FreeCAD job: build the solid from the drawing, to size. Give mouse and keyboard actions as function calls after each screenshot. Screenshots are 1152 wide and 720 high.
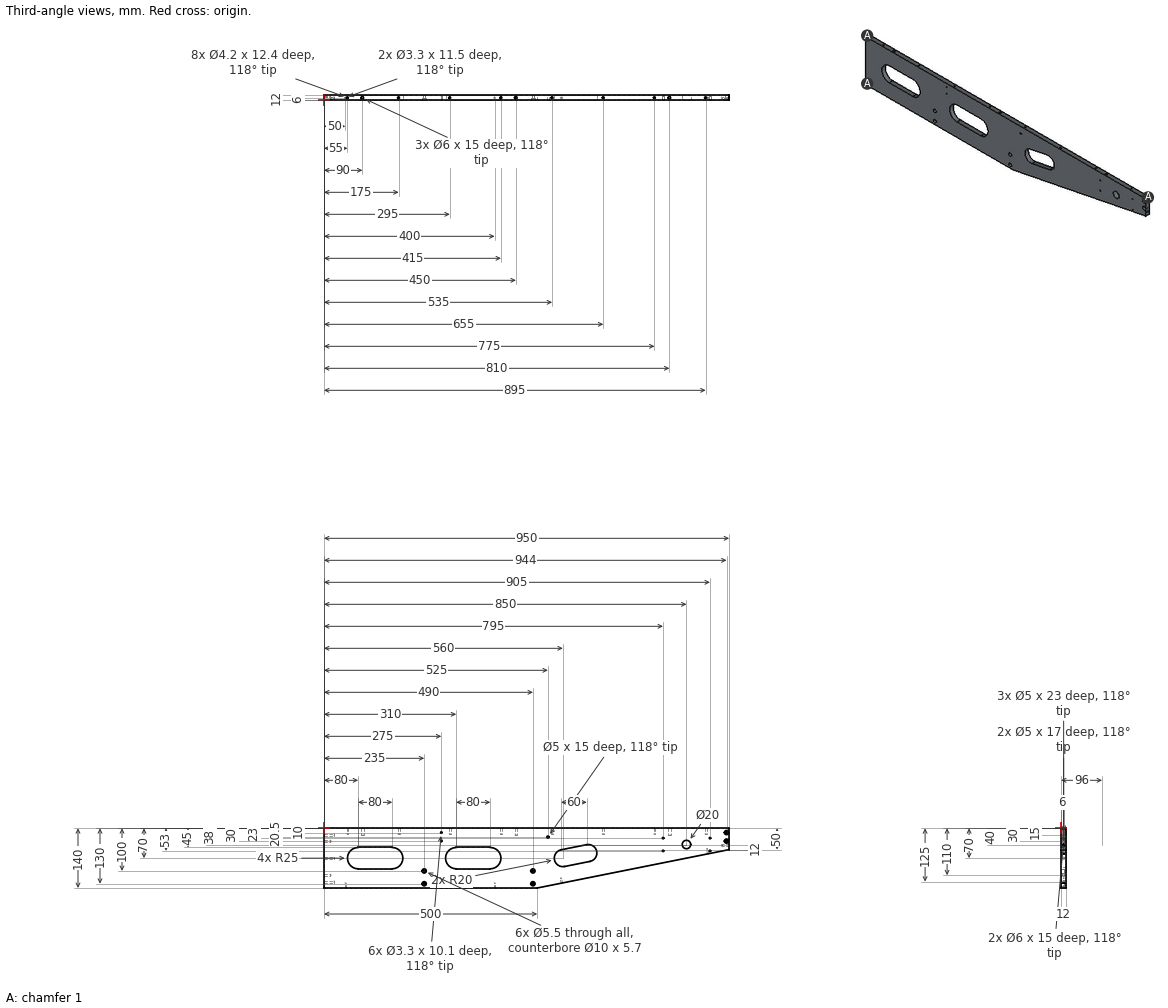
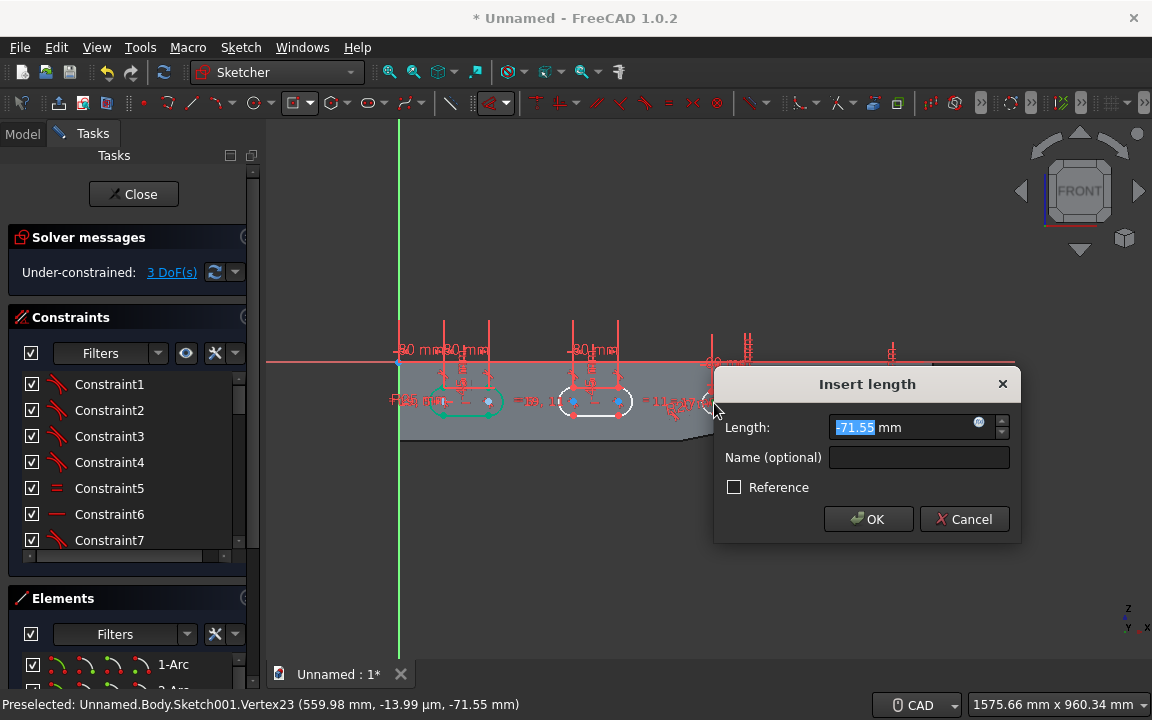
text(-70)
key(Return)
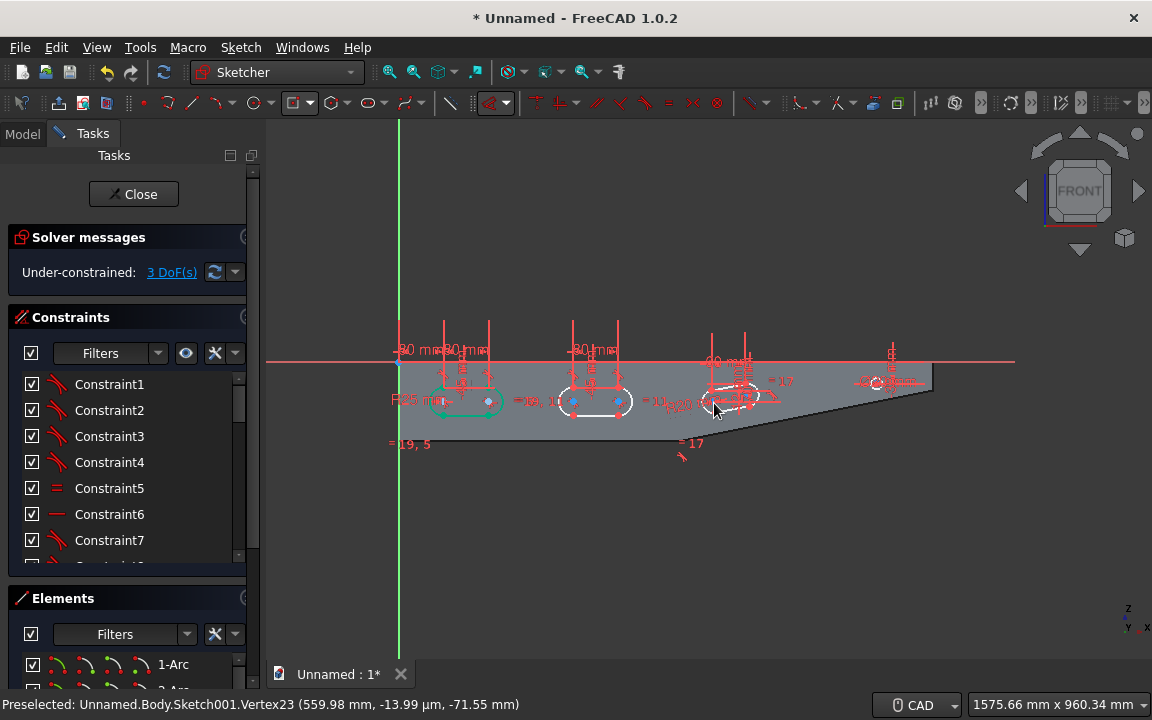
click(877, 384)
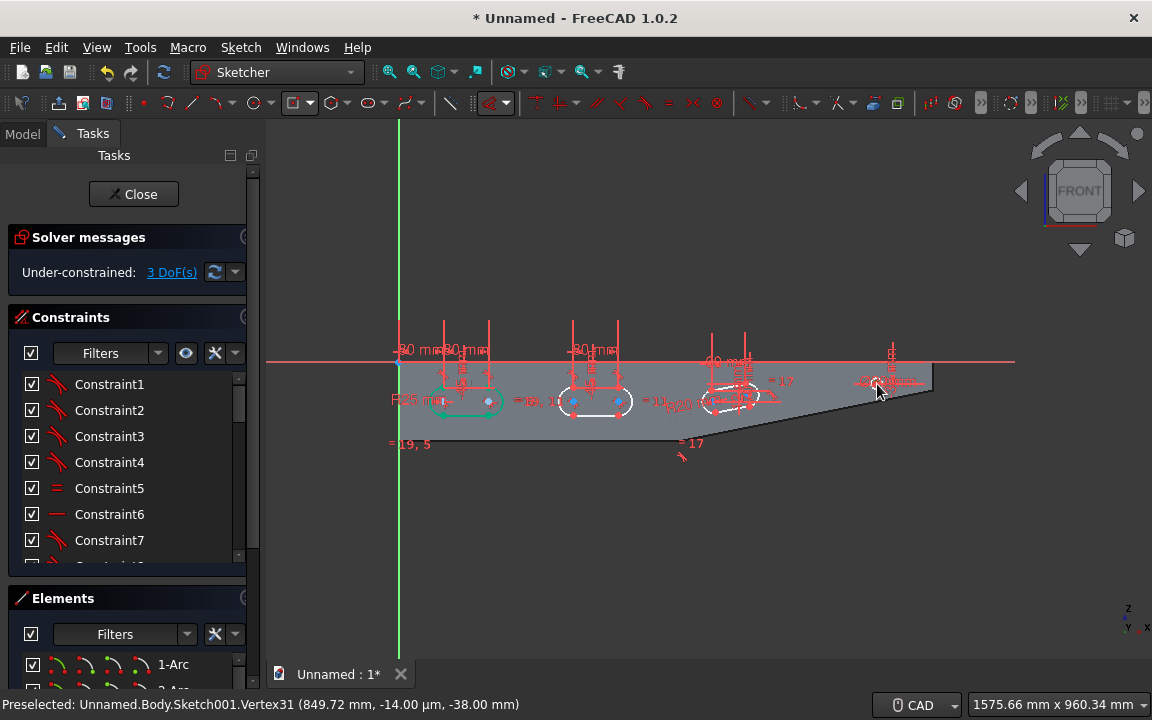
key(l)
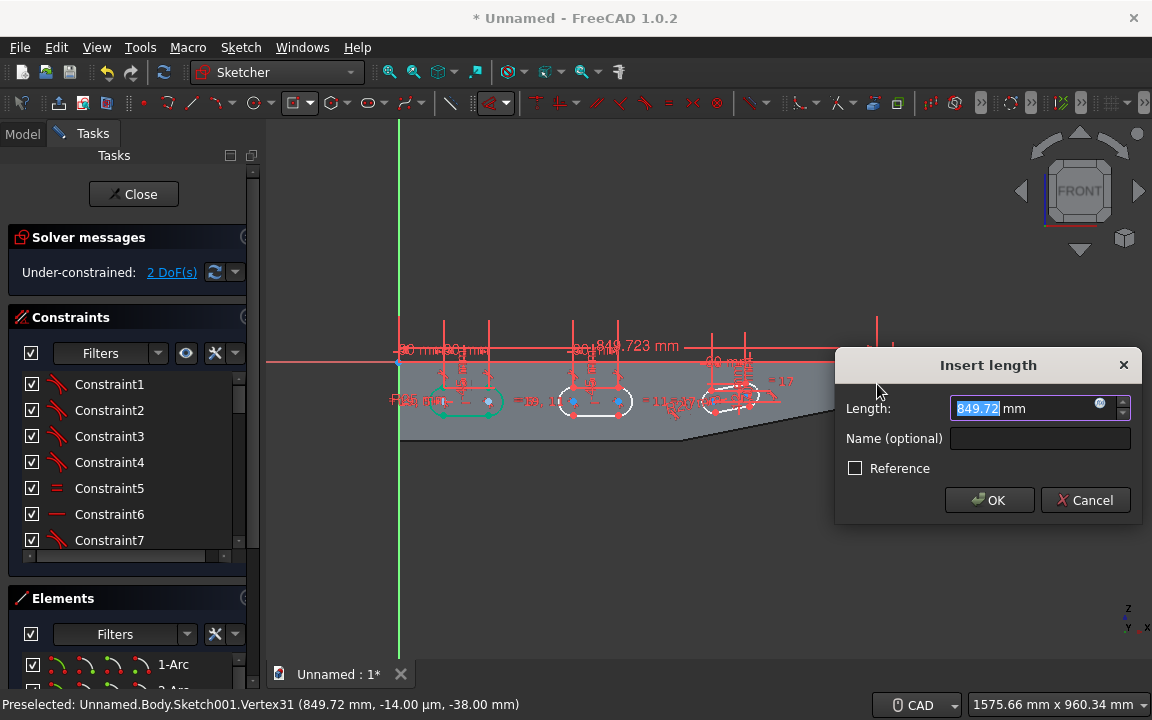
text(850)
key(Return)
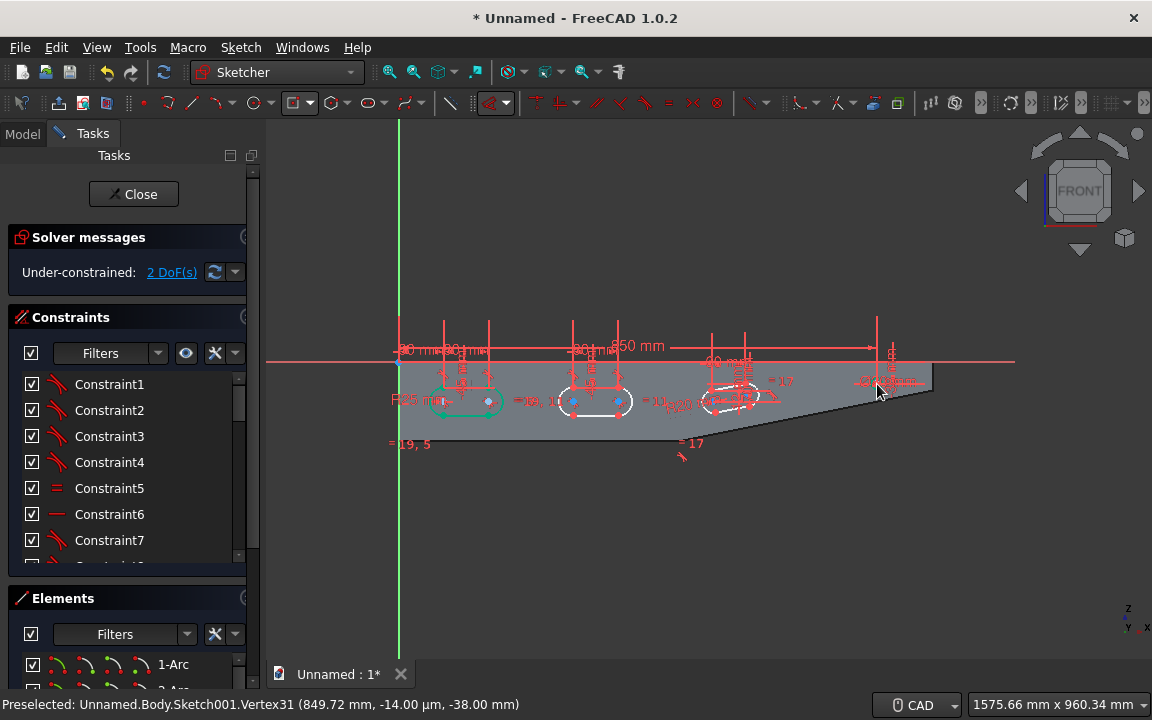
click(573, 388)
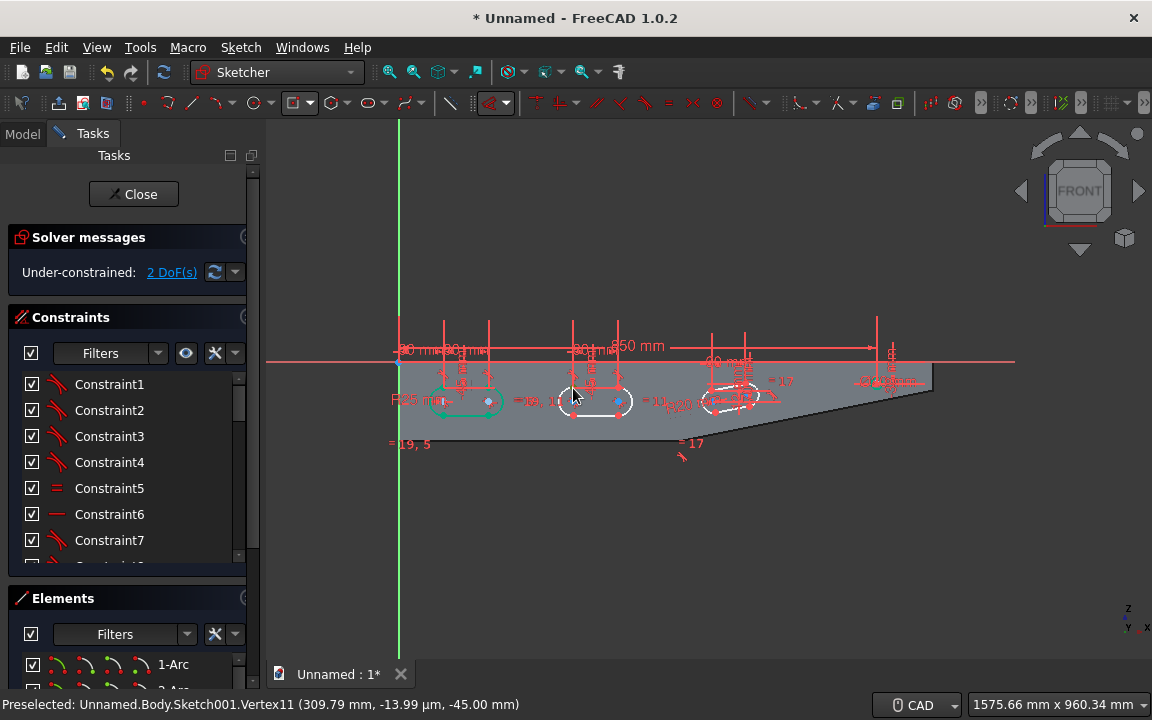
key(l)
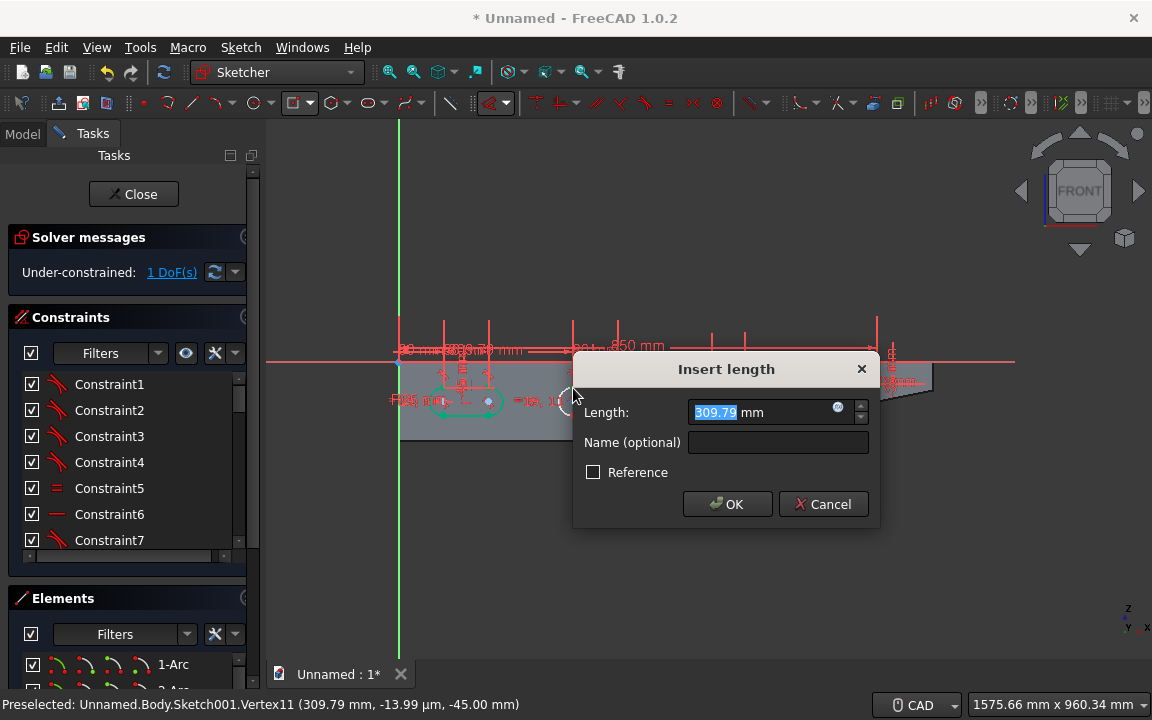
text(310)
key(Return)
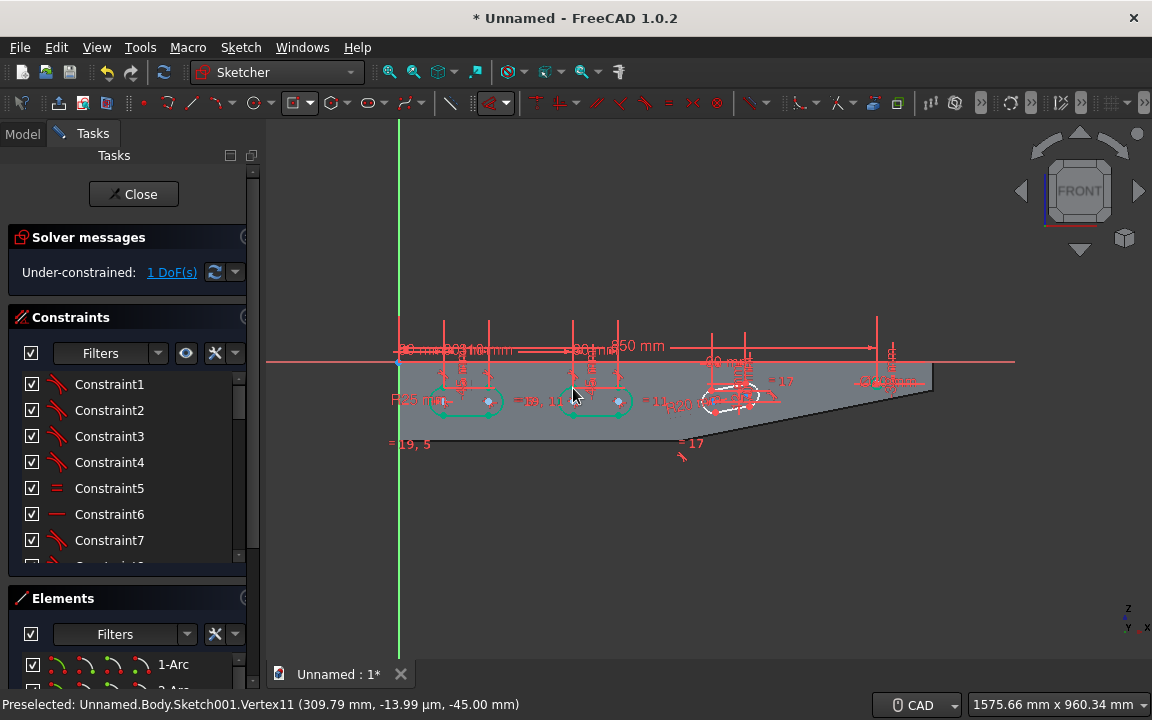
click(714, 402)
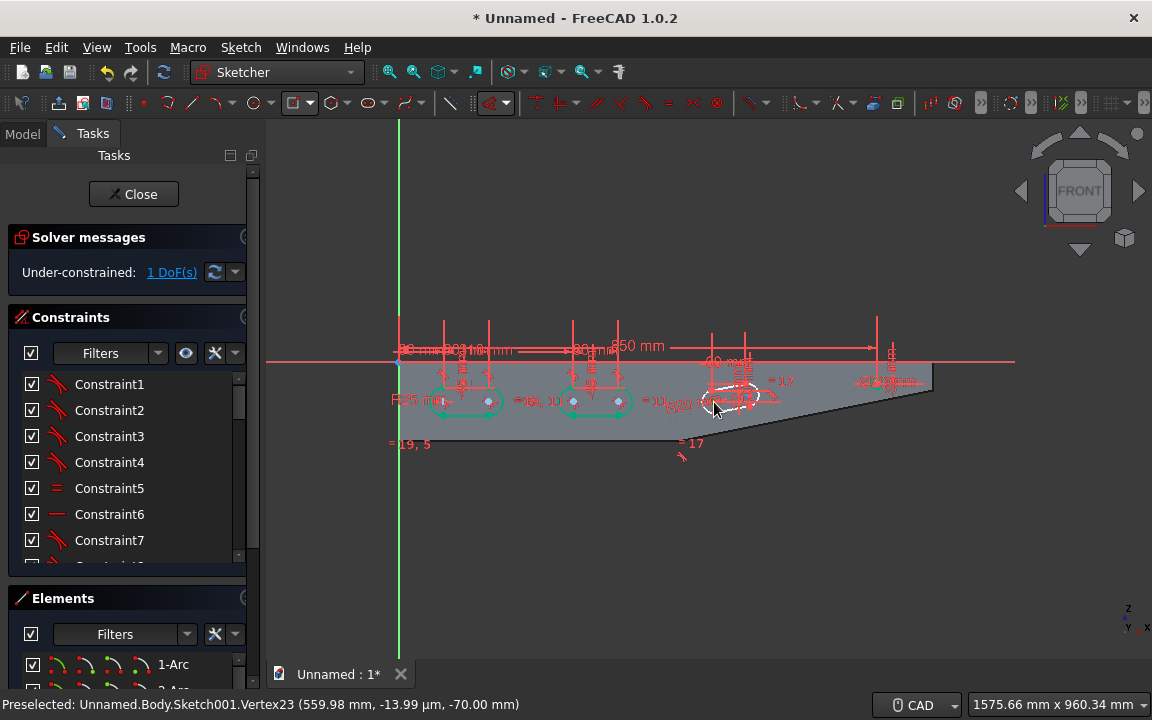
key(l)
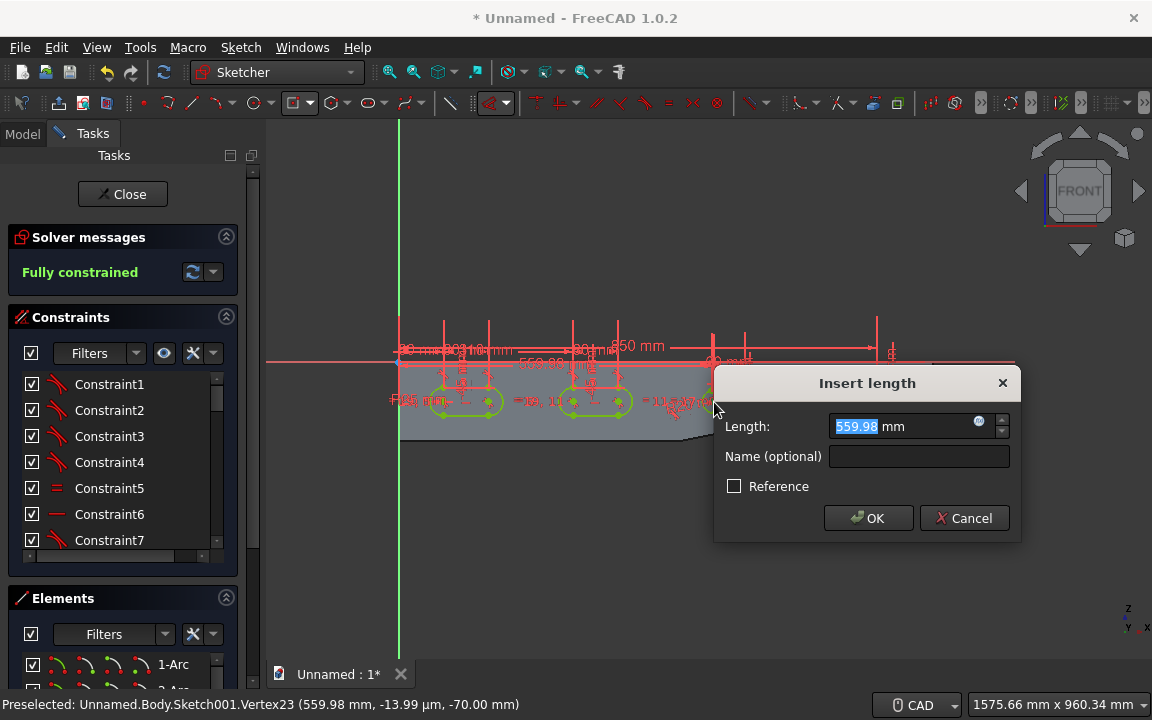
text(560)
key(Return)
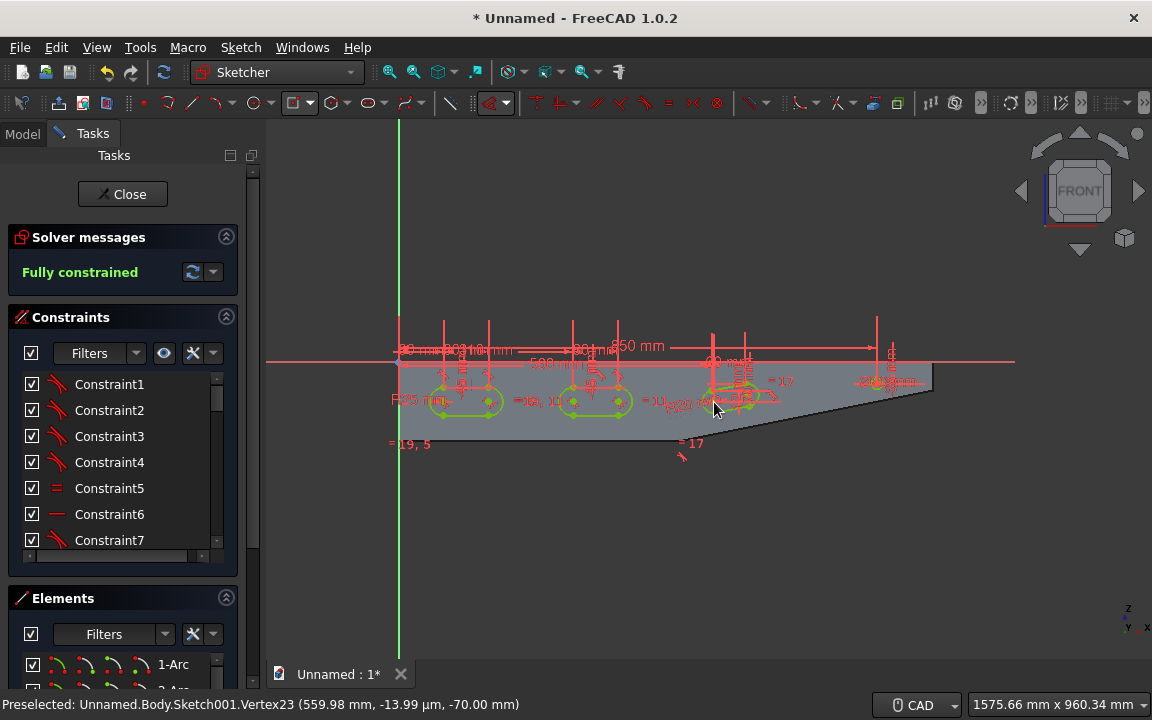
click(123, 194)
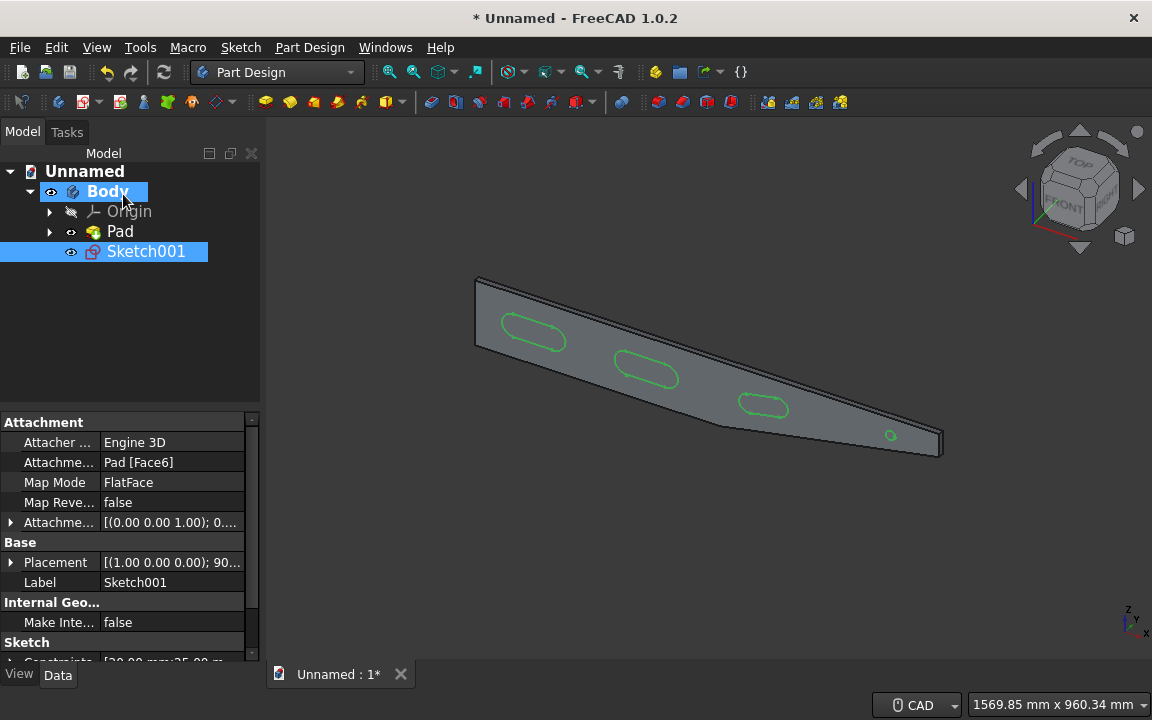
click(432, 102)